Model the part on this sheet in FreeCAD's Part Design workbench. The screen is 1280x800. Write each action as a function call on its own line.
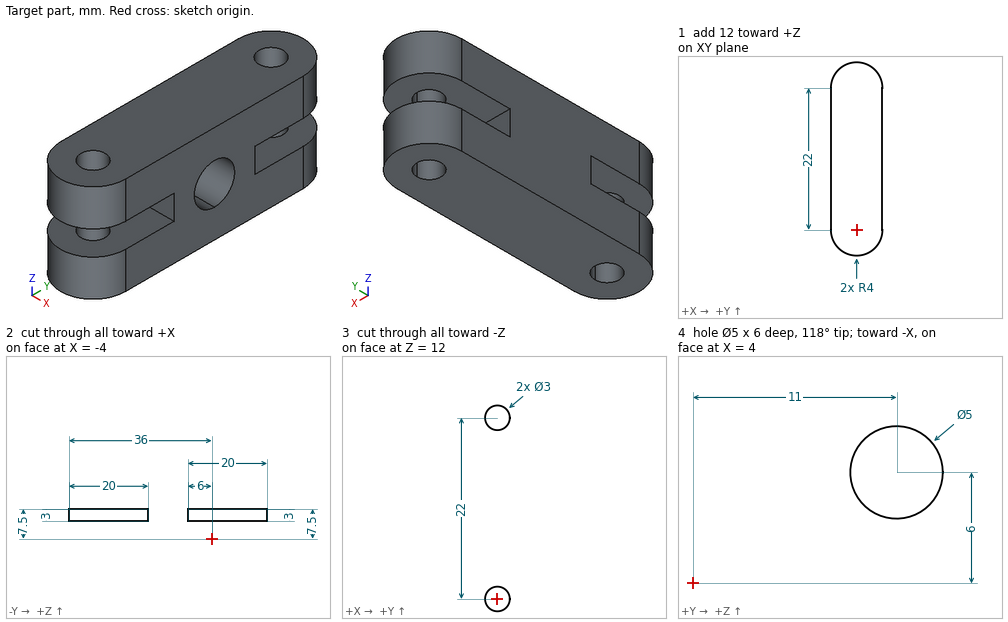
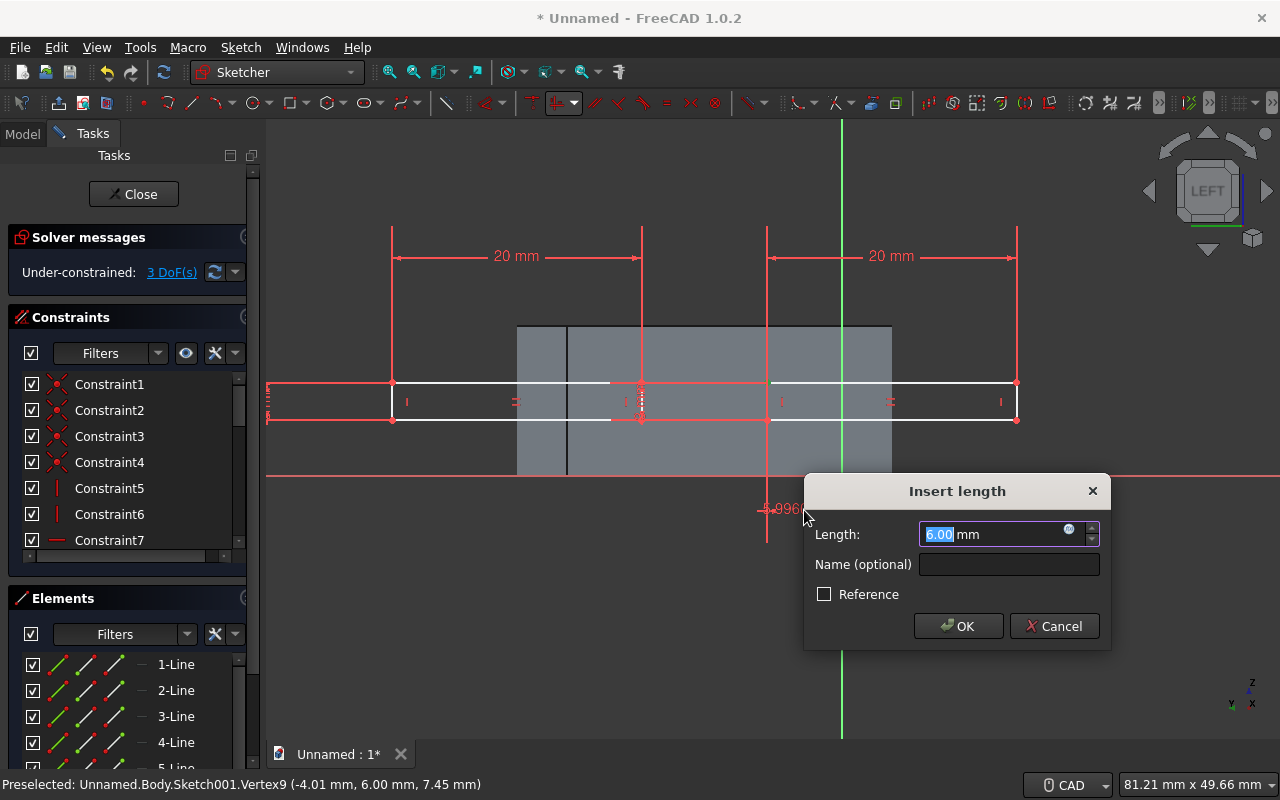
text(6)
key(Return)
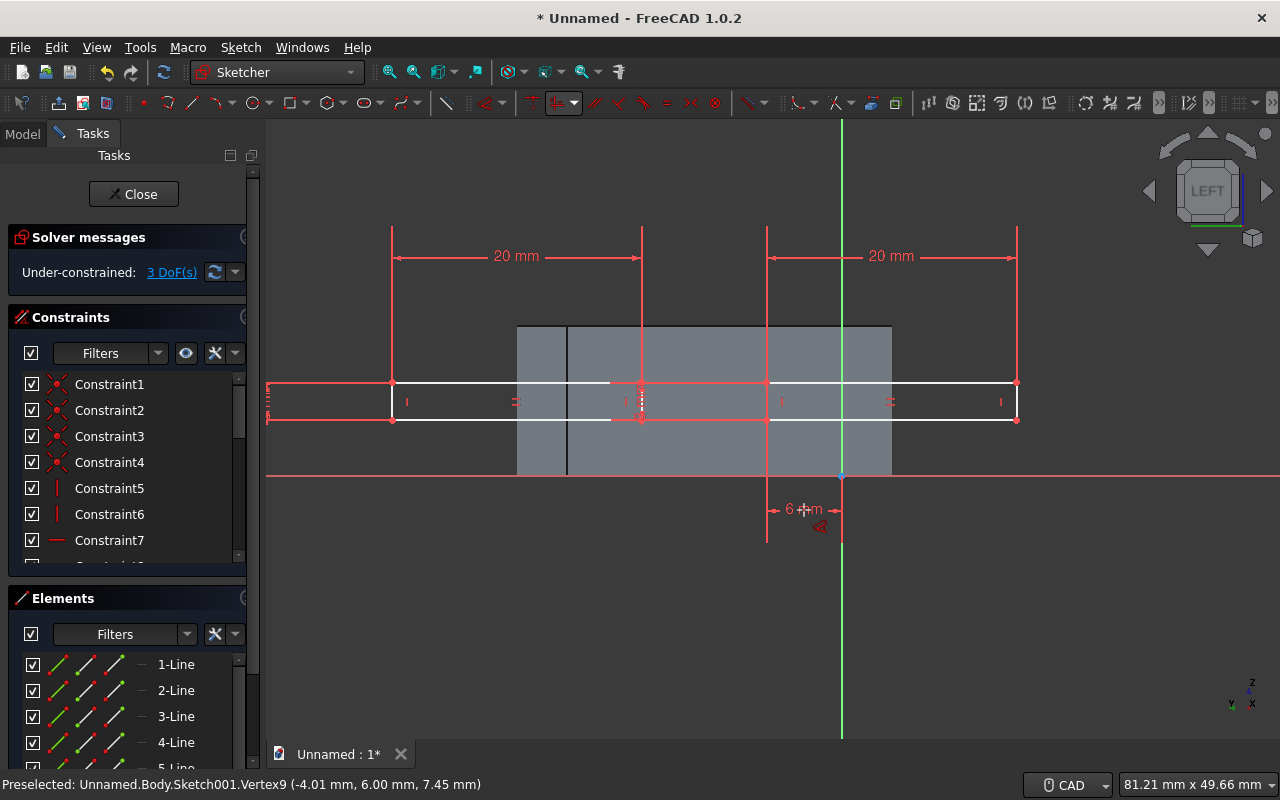
click(392, 383)
click(617, 510)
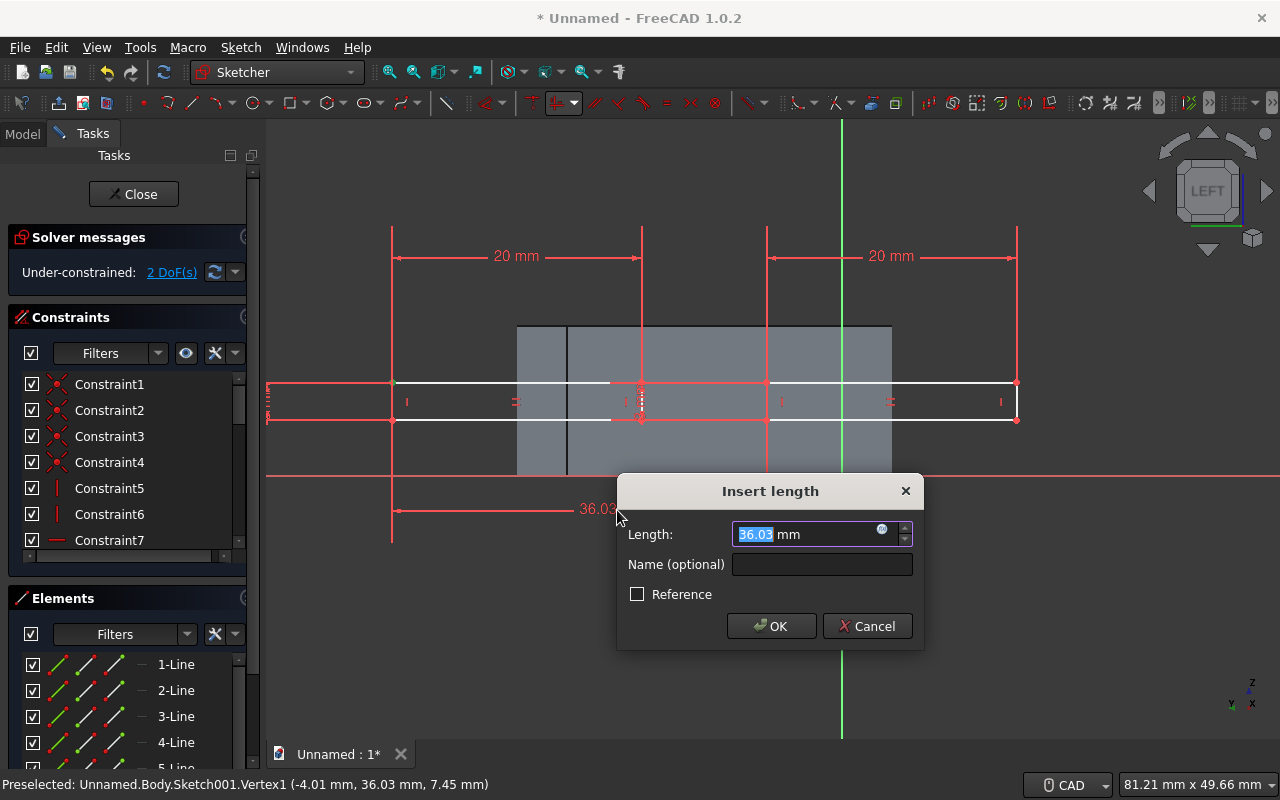
text(36)
key(Return)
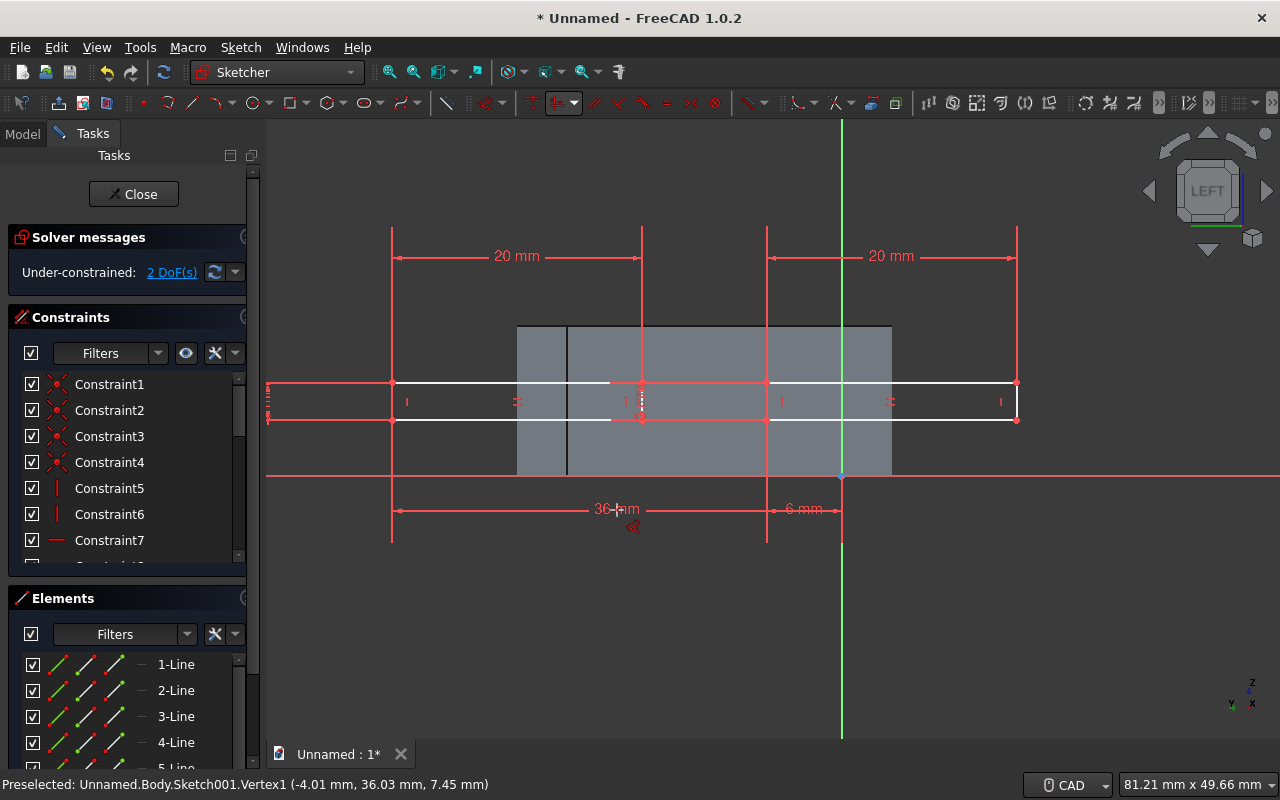
click(392, 383)
click(358, 430)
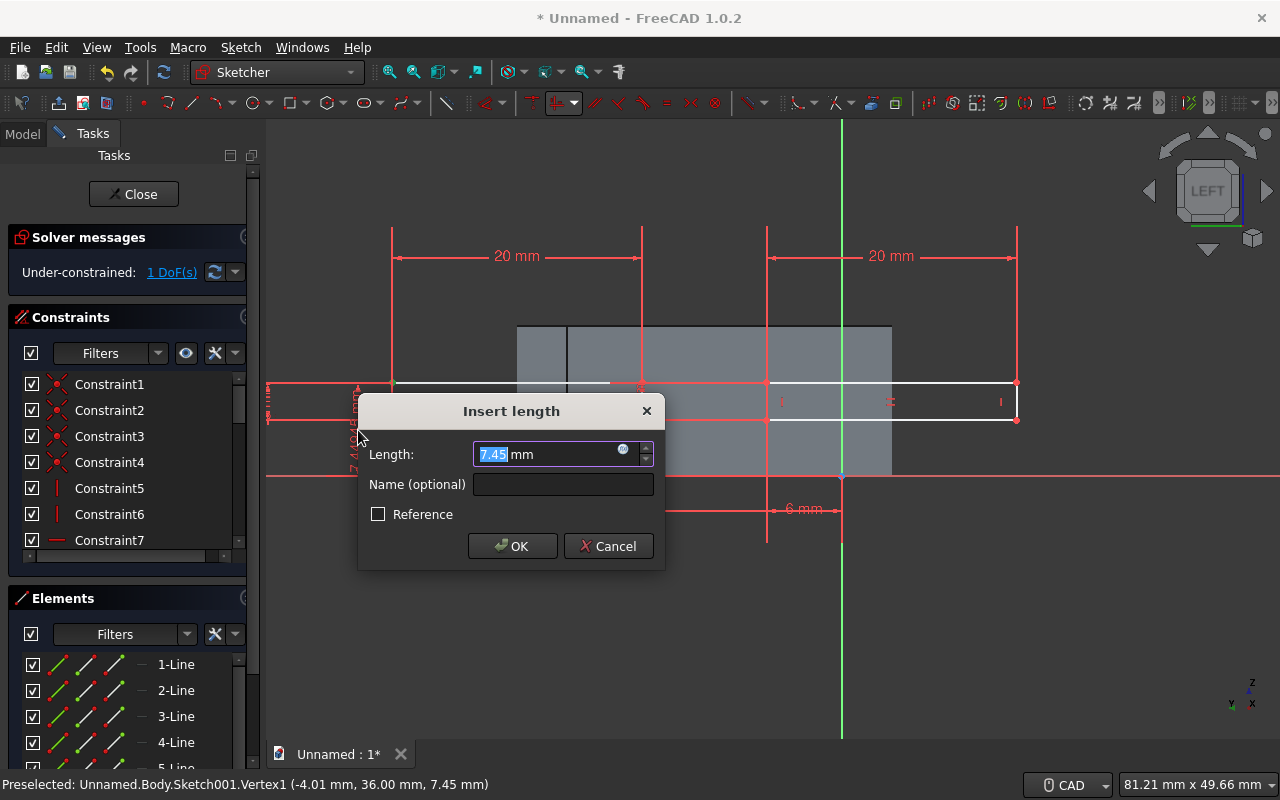
text(7.5)
key(Return)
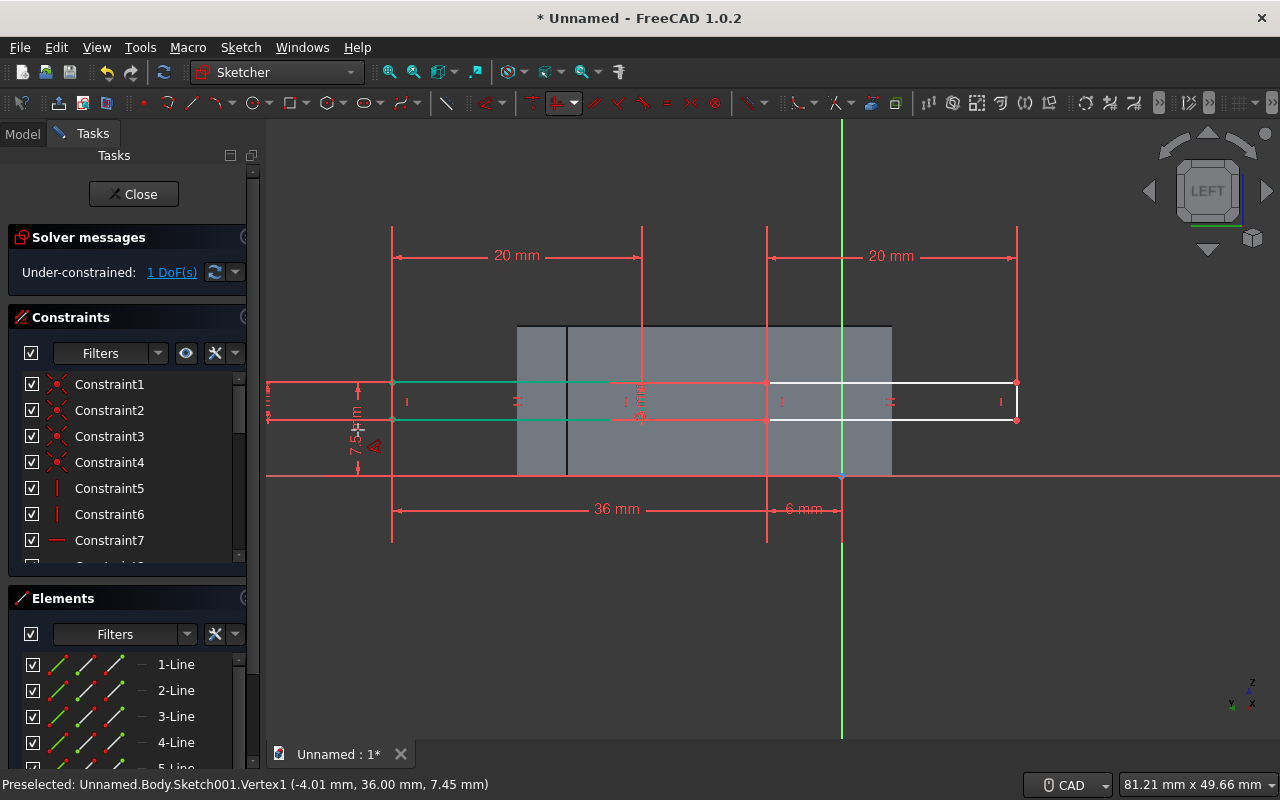
click(767, 383)
click(876, 451)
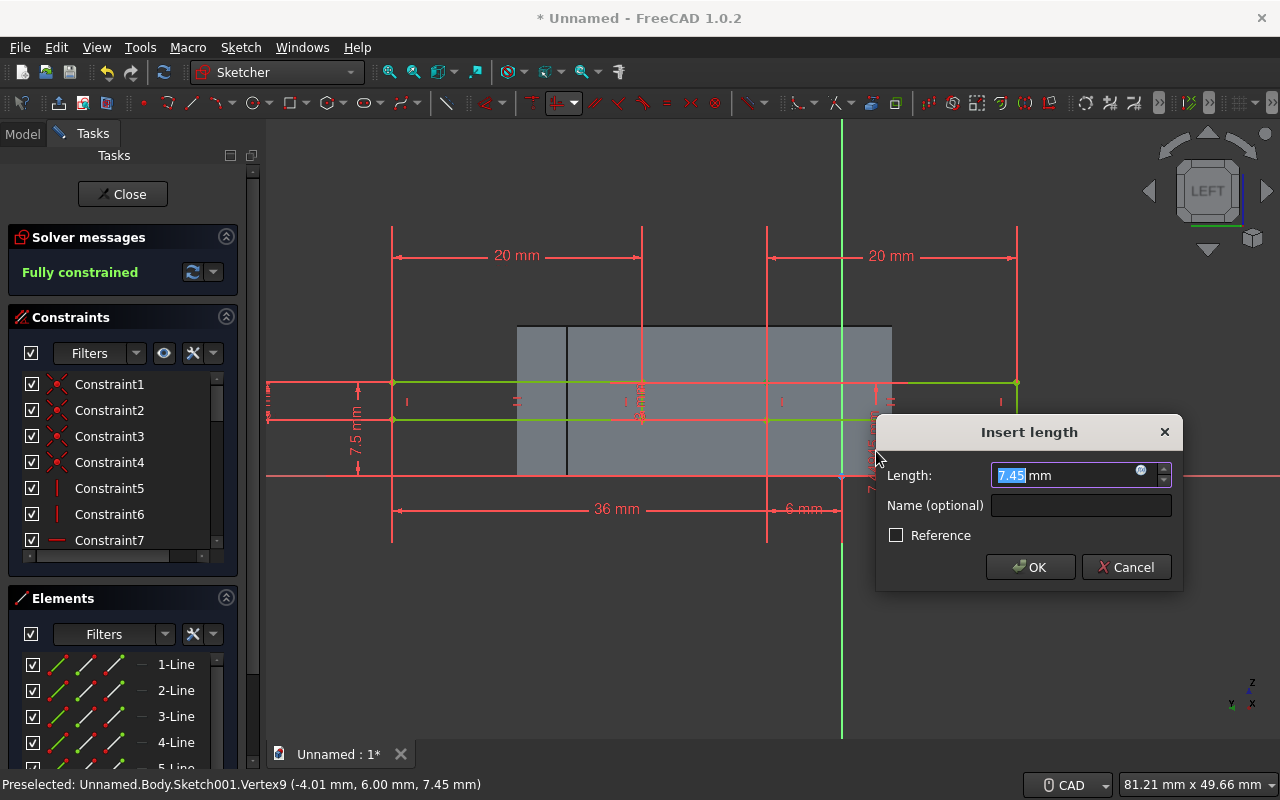
text(7.5)
key(Return)
key(Escape)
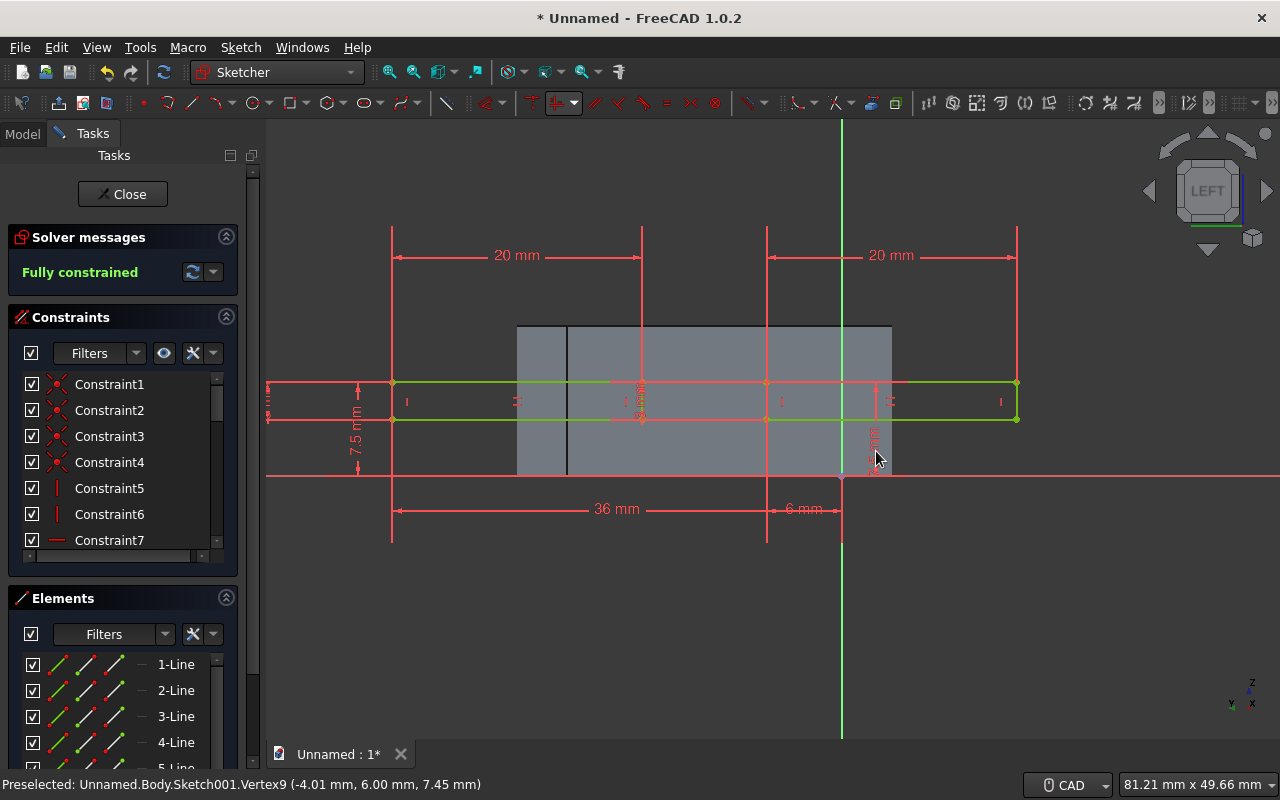
click(123, 194)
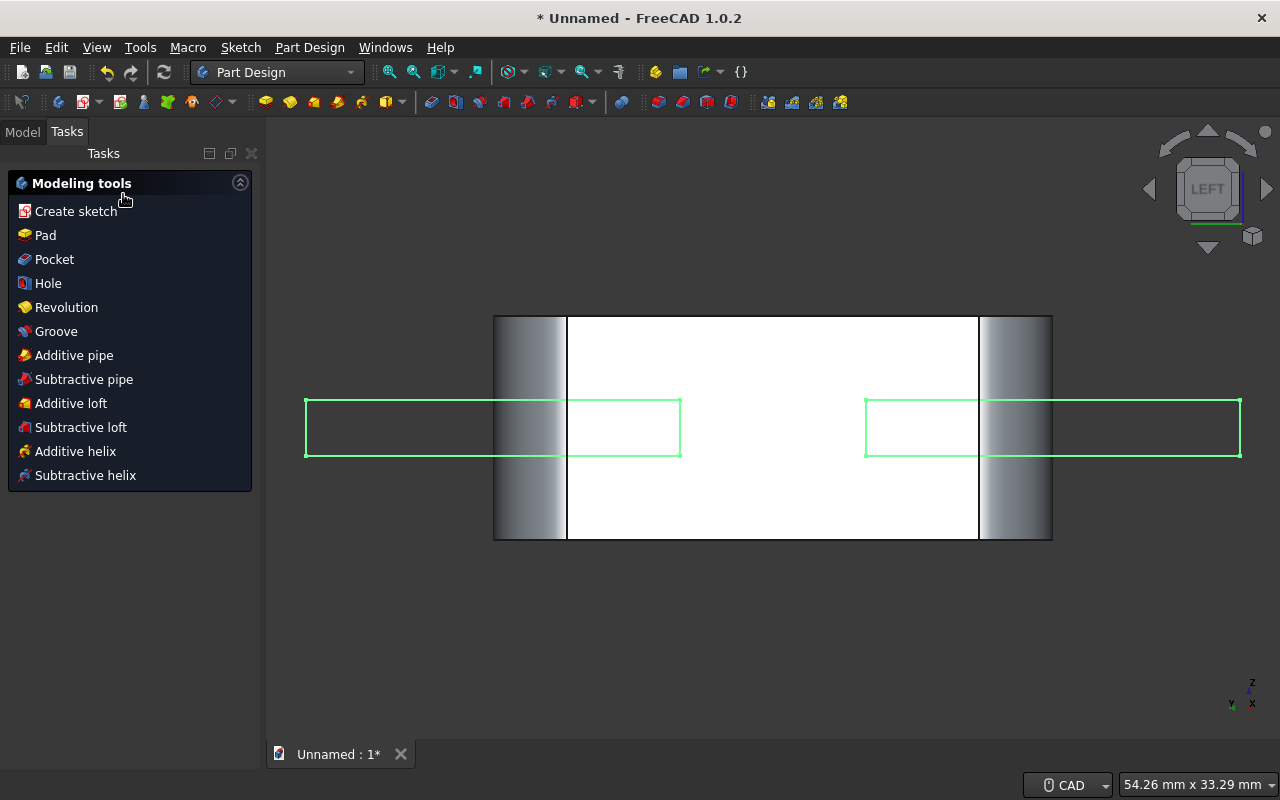
click(432, 102)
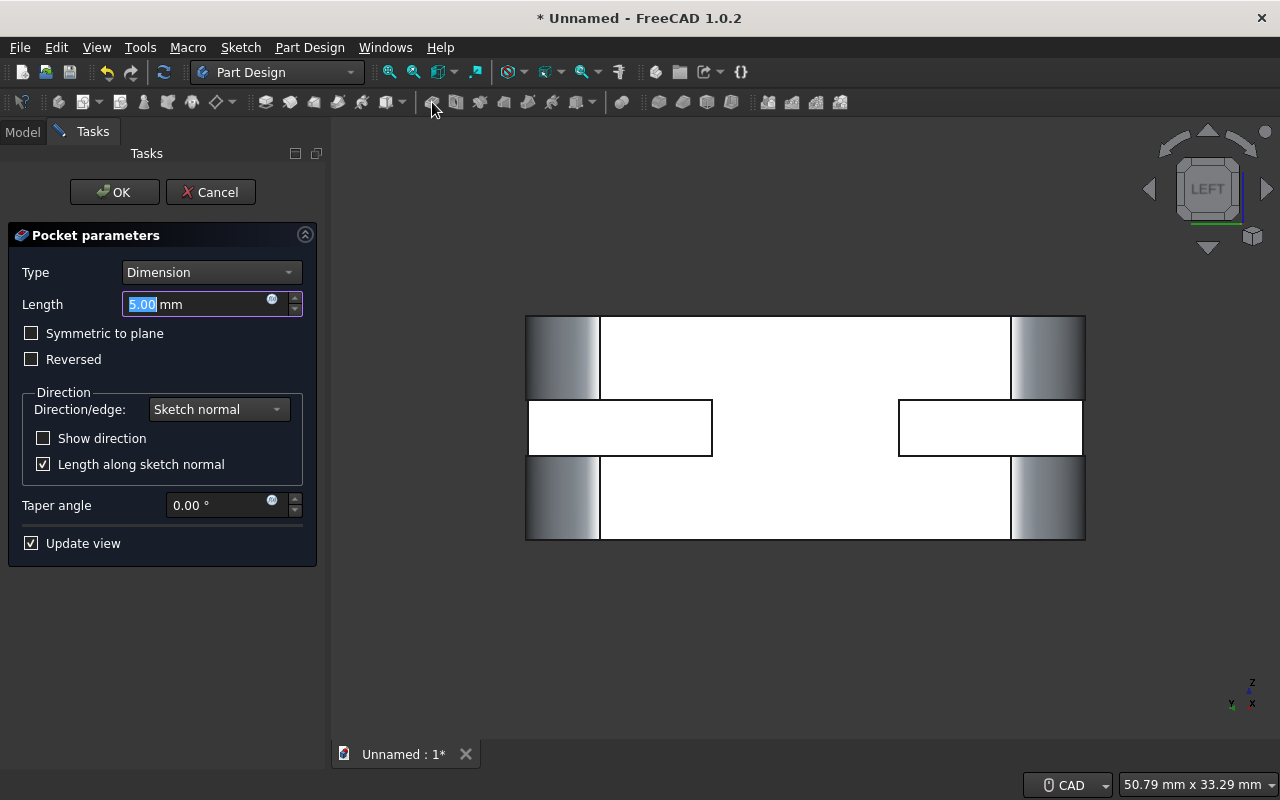
click(212, 272)